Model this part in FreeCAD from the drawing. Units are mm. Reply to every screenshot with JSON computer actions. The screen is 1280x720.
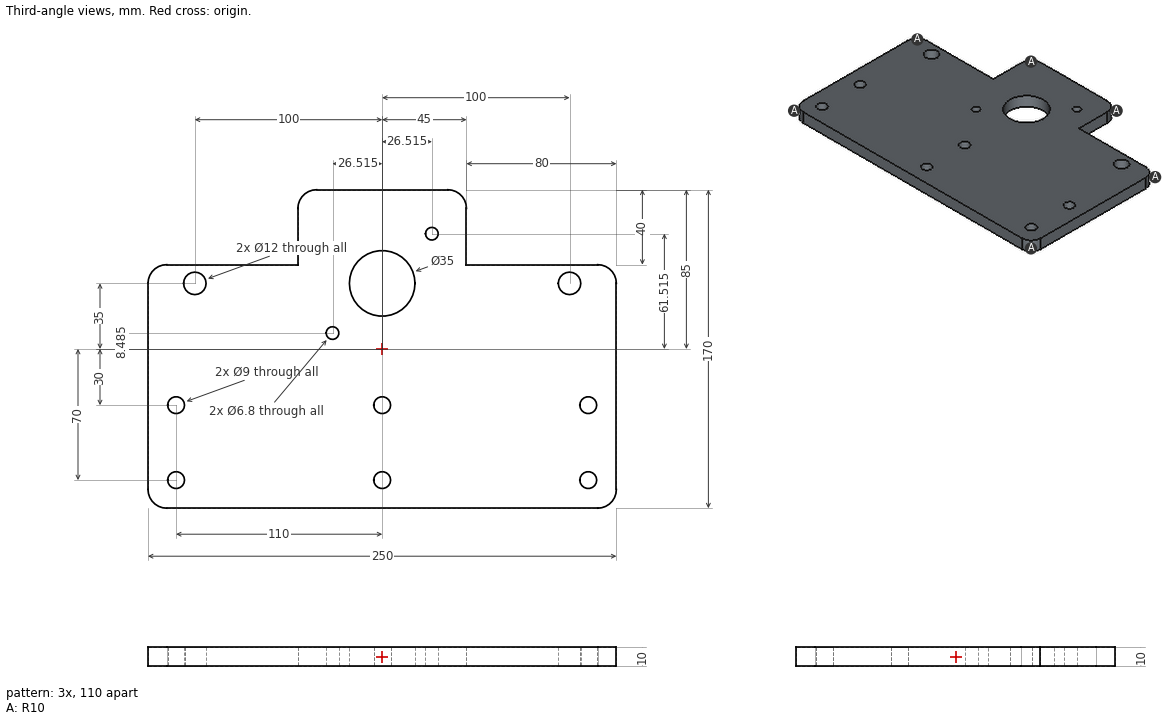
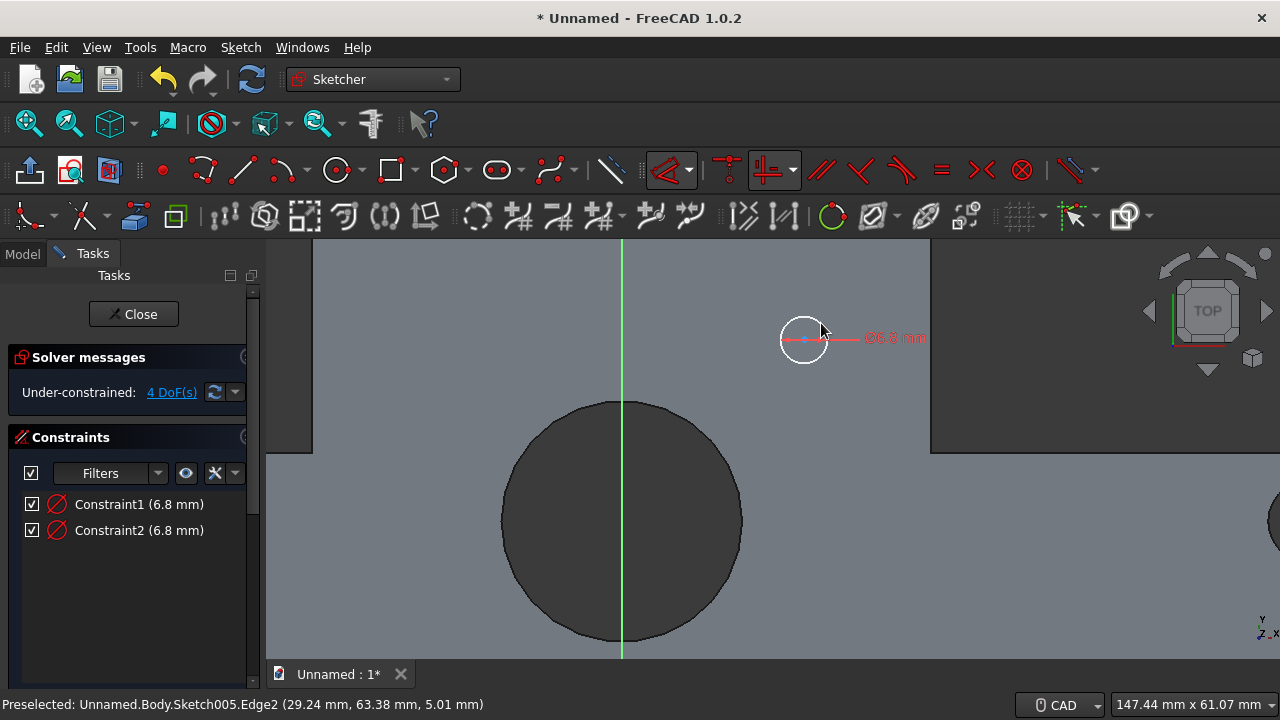
{"action": "scroll", "coordinate": [805, 340], "scroll_direction": "down", "scroll_amount": 3}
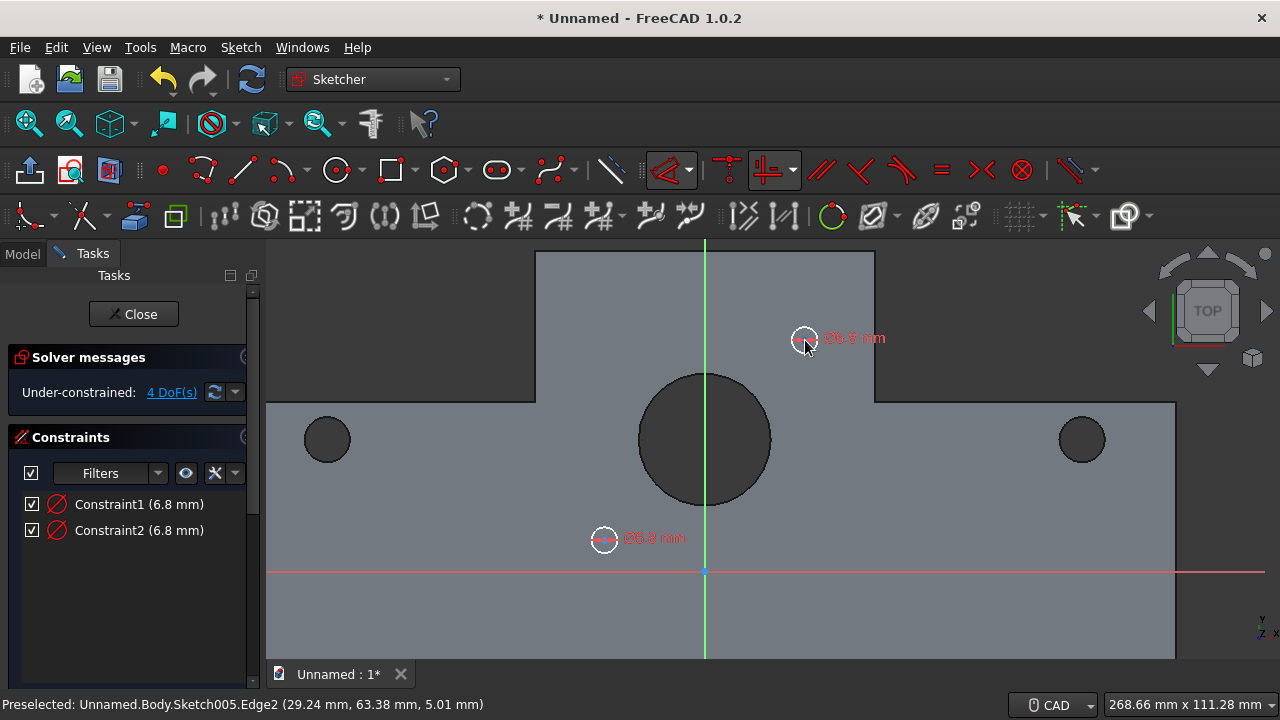
{"action": "scroll", "coordinate": [605, 540], "scroll_direction": "up", "scroll_amount": 2}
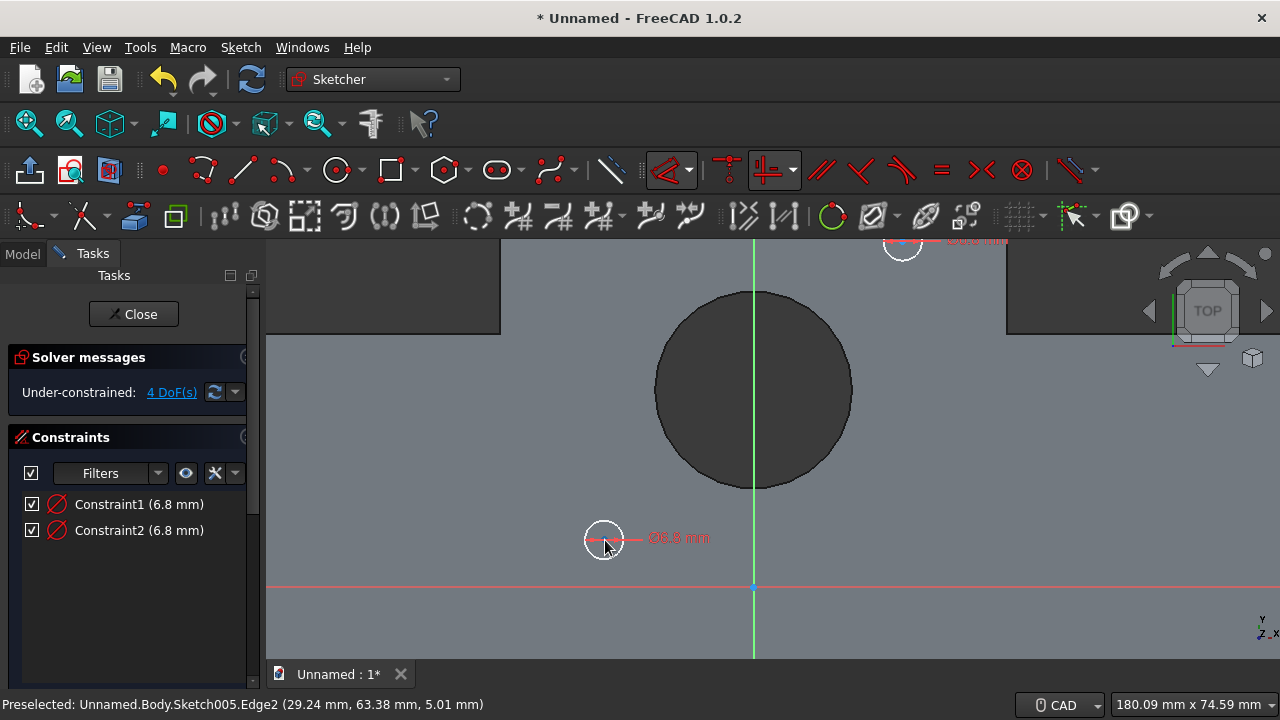
{"action": "left_click", "coordinate": [604, 540]}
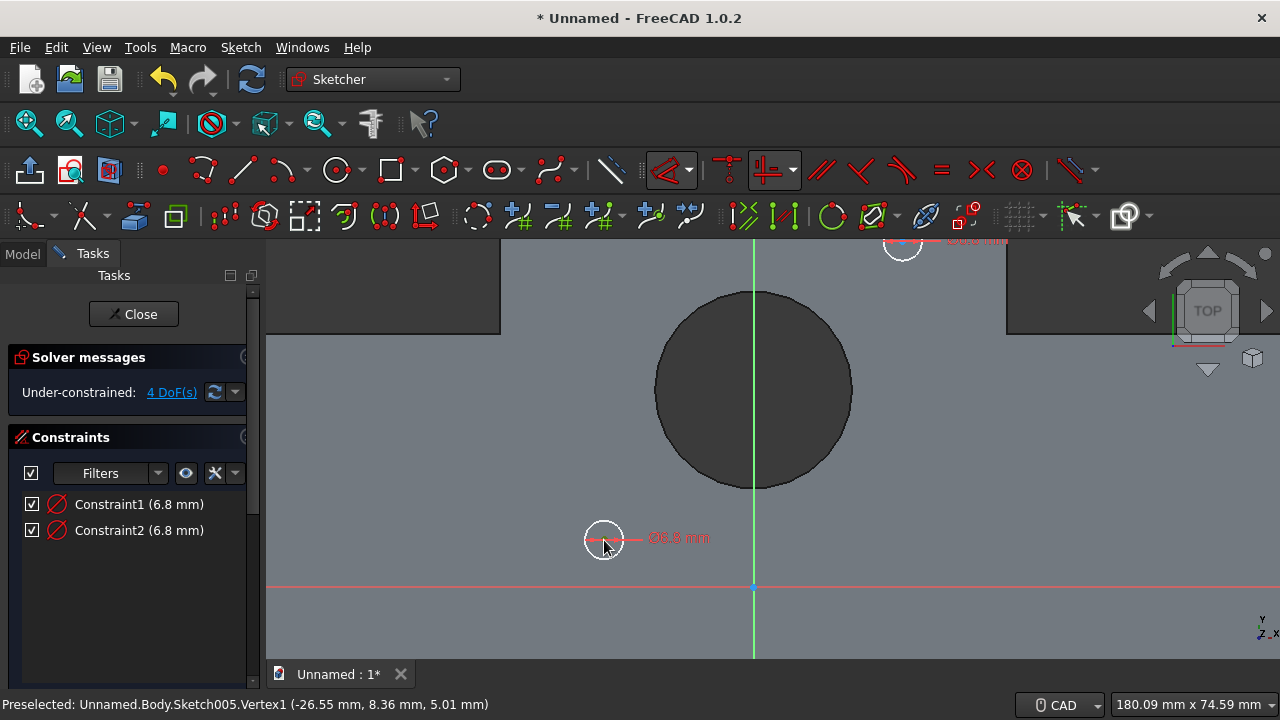
{"action": "left_click", "coordinate": [692, 170]}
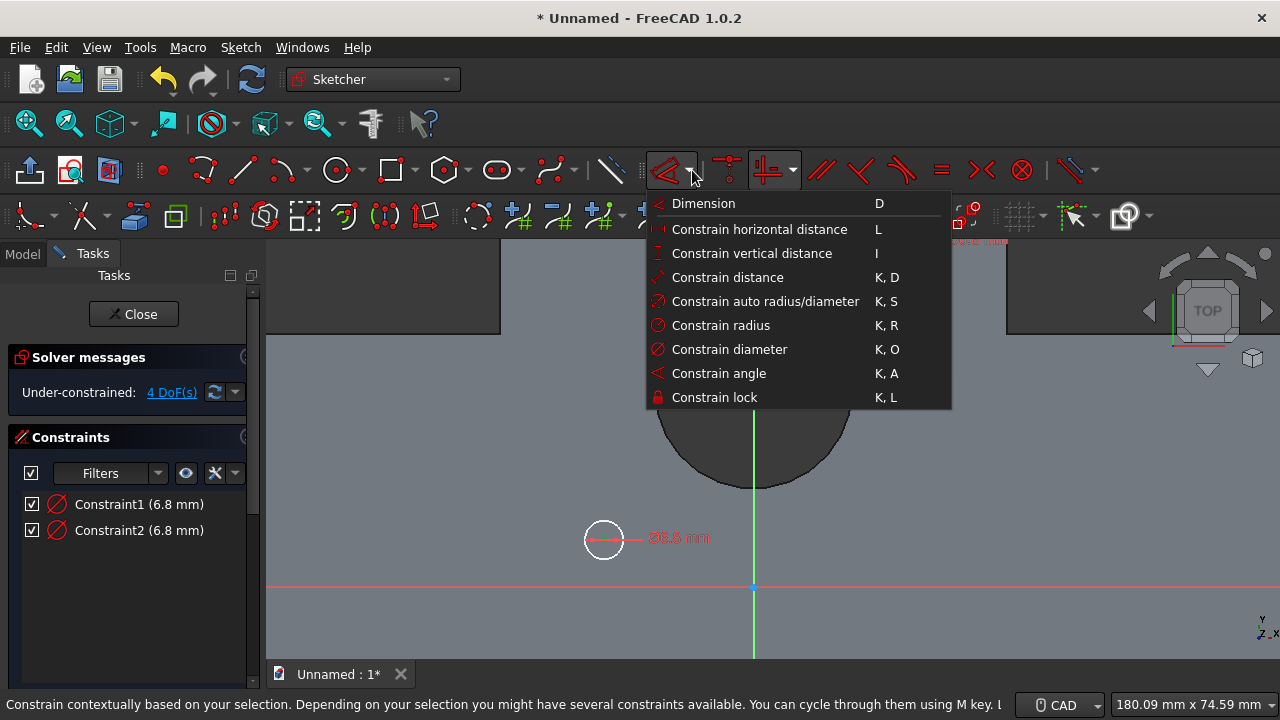
{"action": "left_click", "coordinate": [799, 253]}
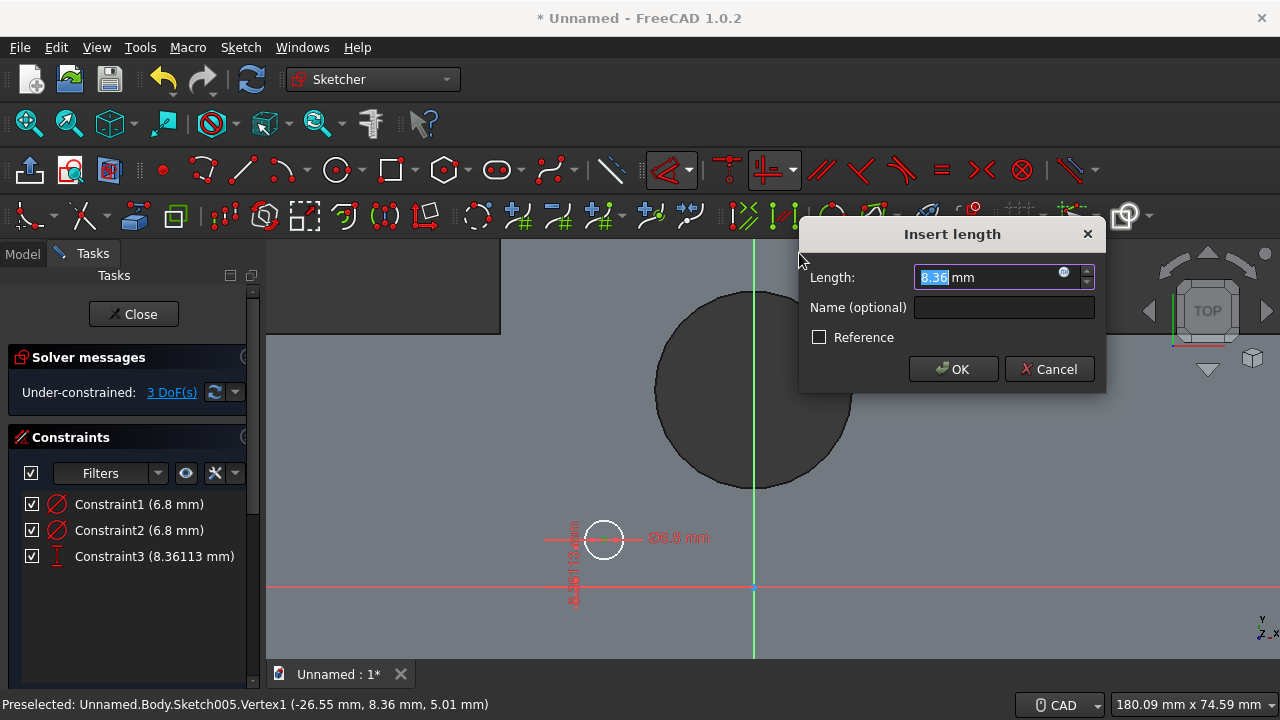
{"action": "type", "text": "8.485"}
{"action": "key", "text": "Return"}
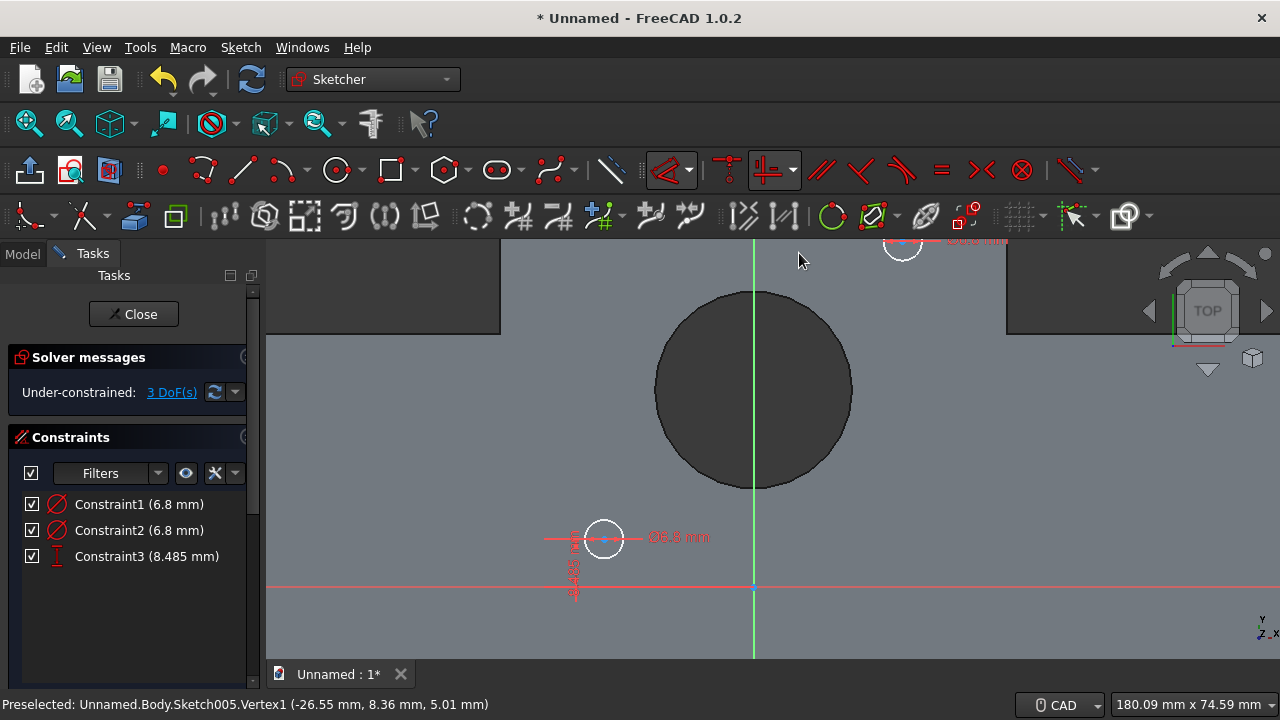
{"action": "left_click", "coordinate": [604, 539]}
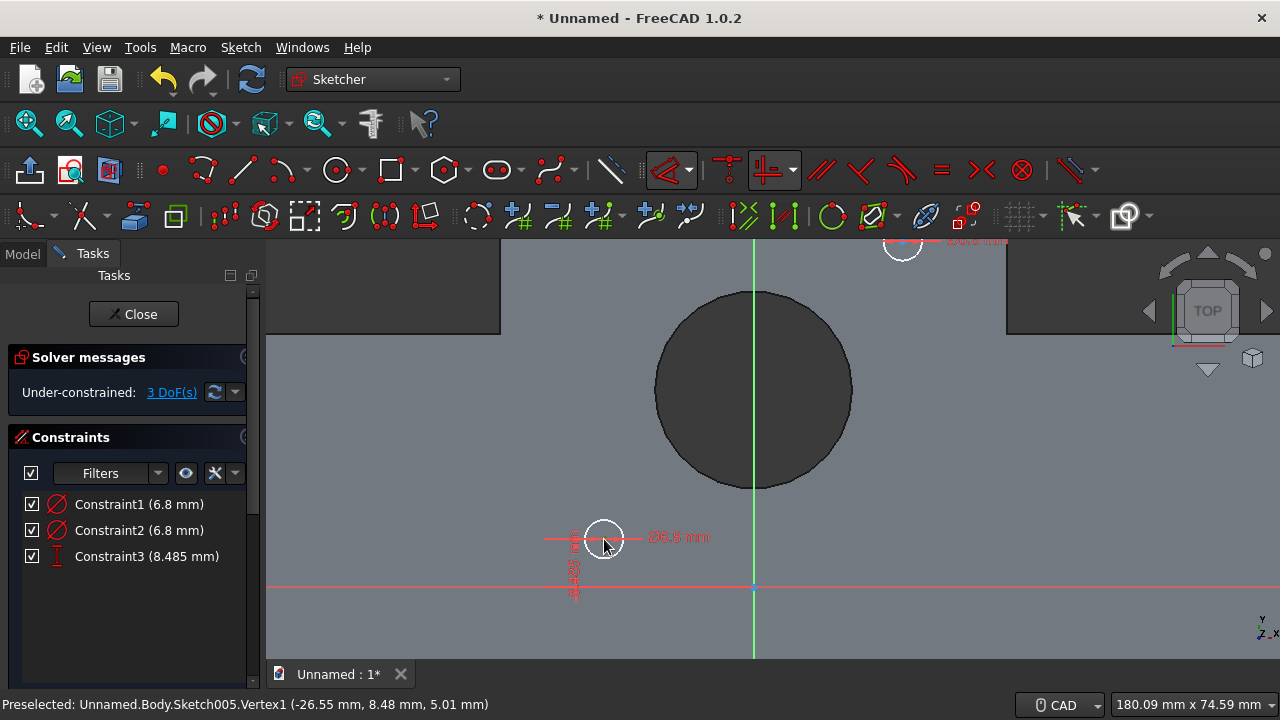
{"action": "key", "text": "l"}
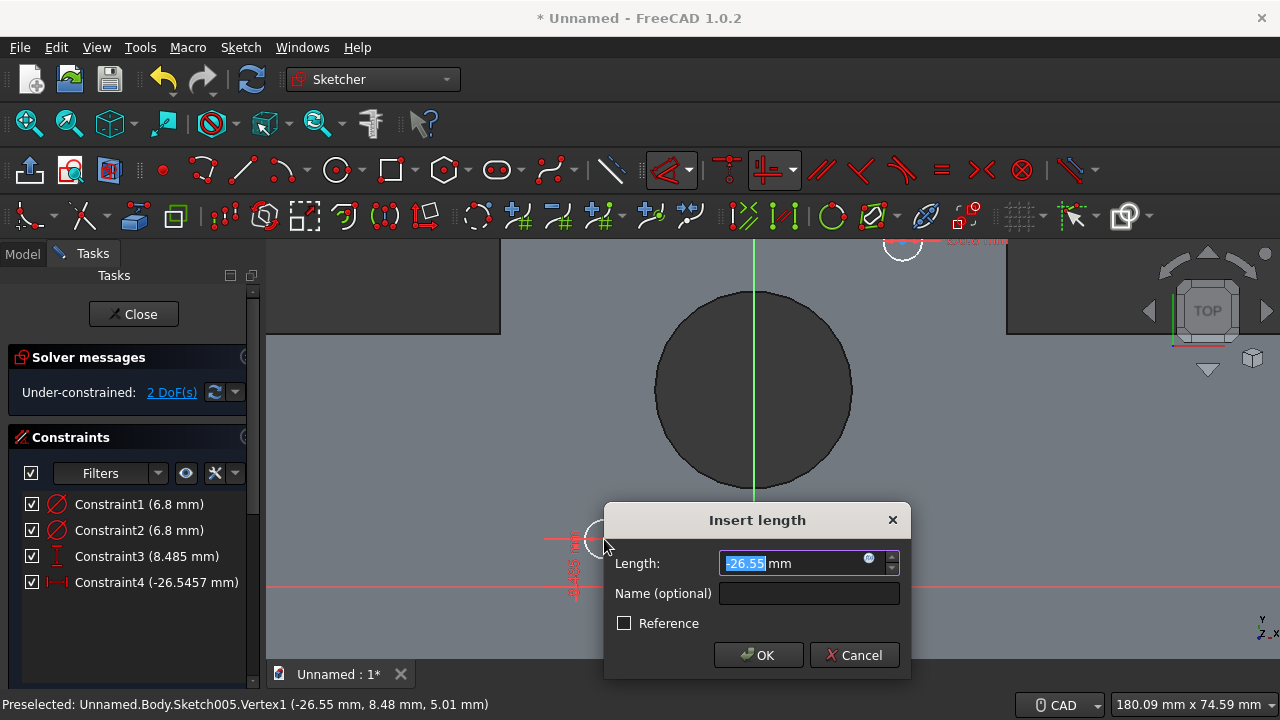
{"action": "type", "text": "-26.515"}
{"action": "key", "text": "Return"}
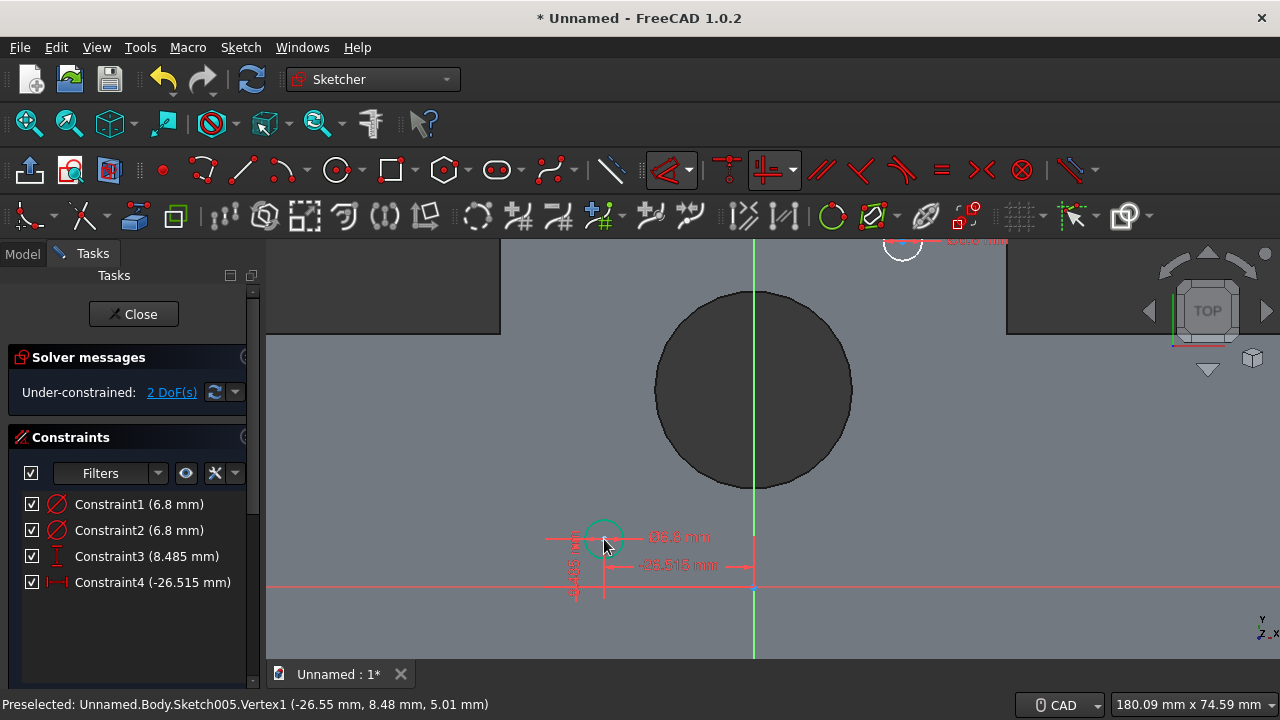
{"action": "scroll", "coordinate": [605, 540], "scroll_direction": "down", "scroll_amount": 2}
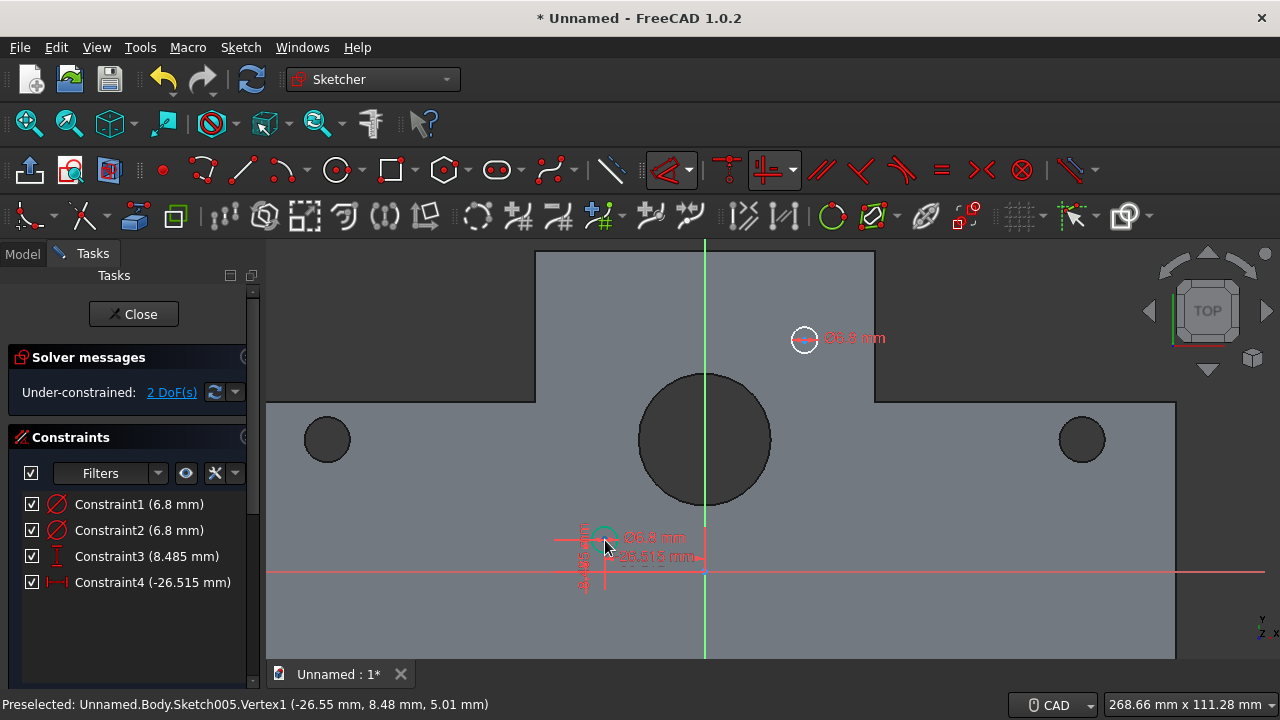
{"action": "left_click", "coordinate": [805, 340]}